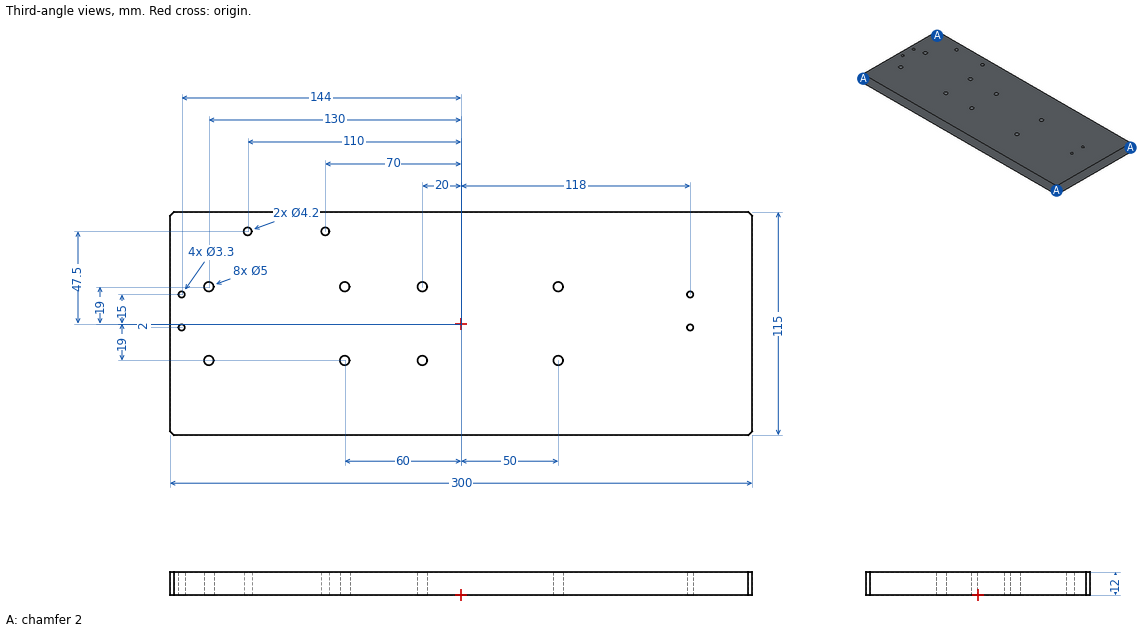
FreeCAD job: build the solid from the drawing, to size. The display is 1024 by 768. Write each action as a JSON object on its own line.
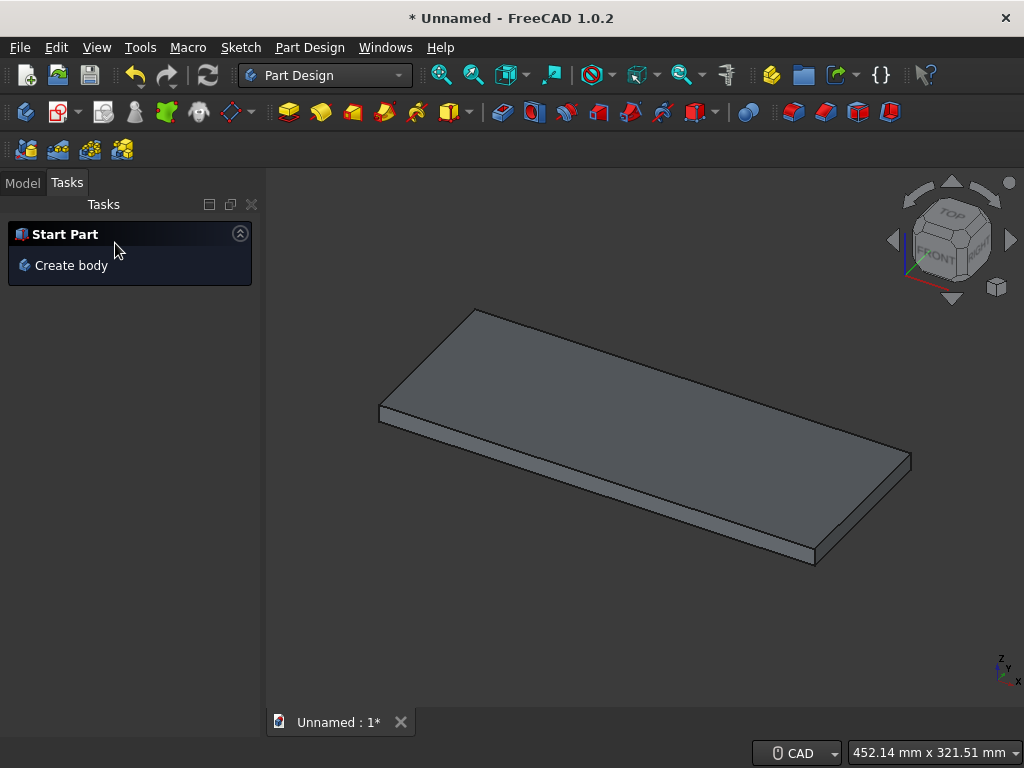
{"action": "left_click", "coordinate": [58, 112]}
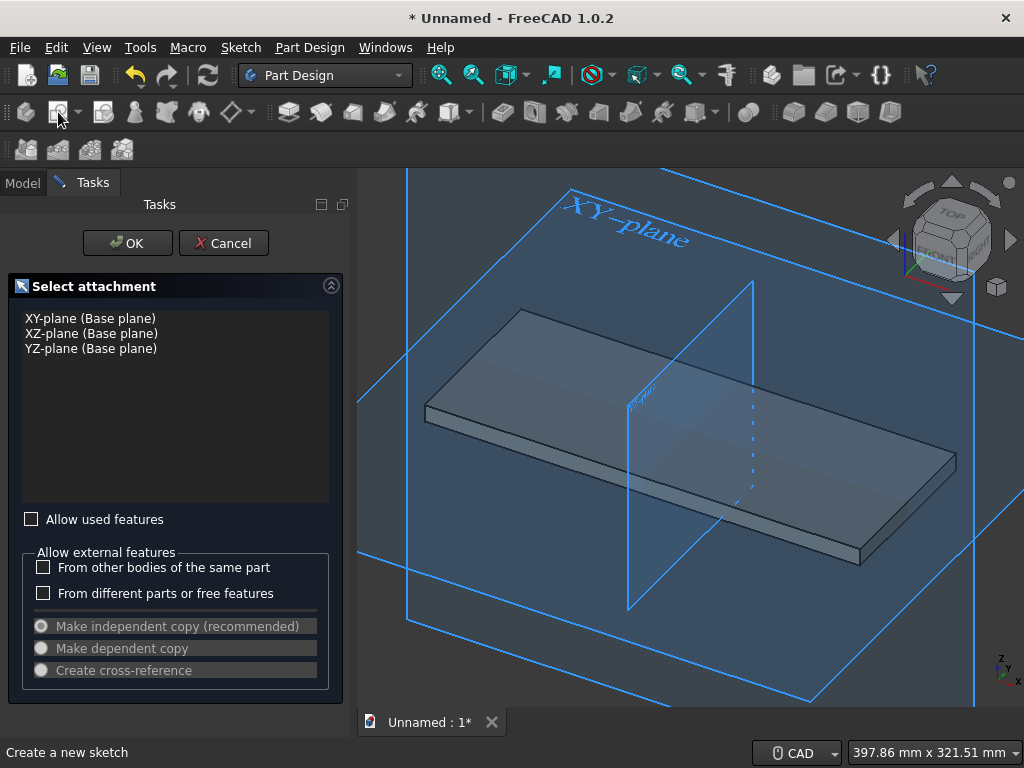
{"action": "left_click", "coordinate": [82, 318]}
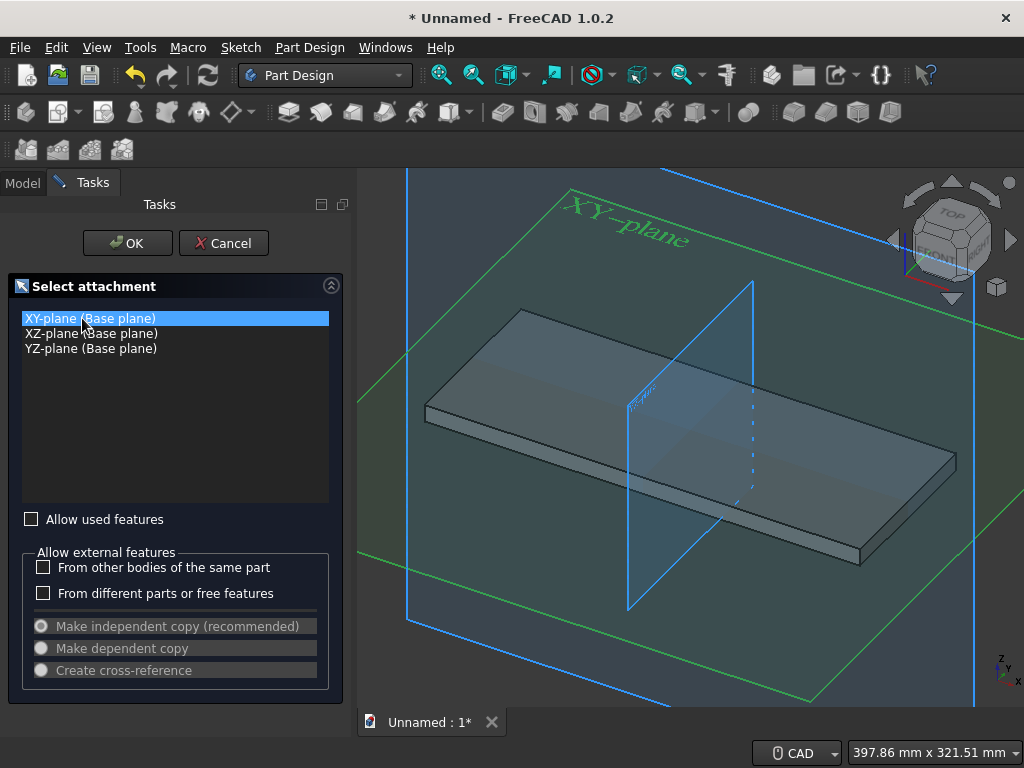
{"action": "left_click", "coordinate": [128, 243]}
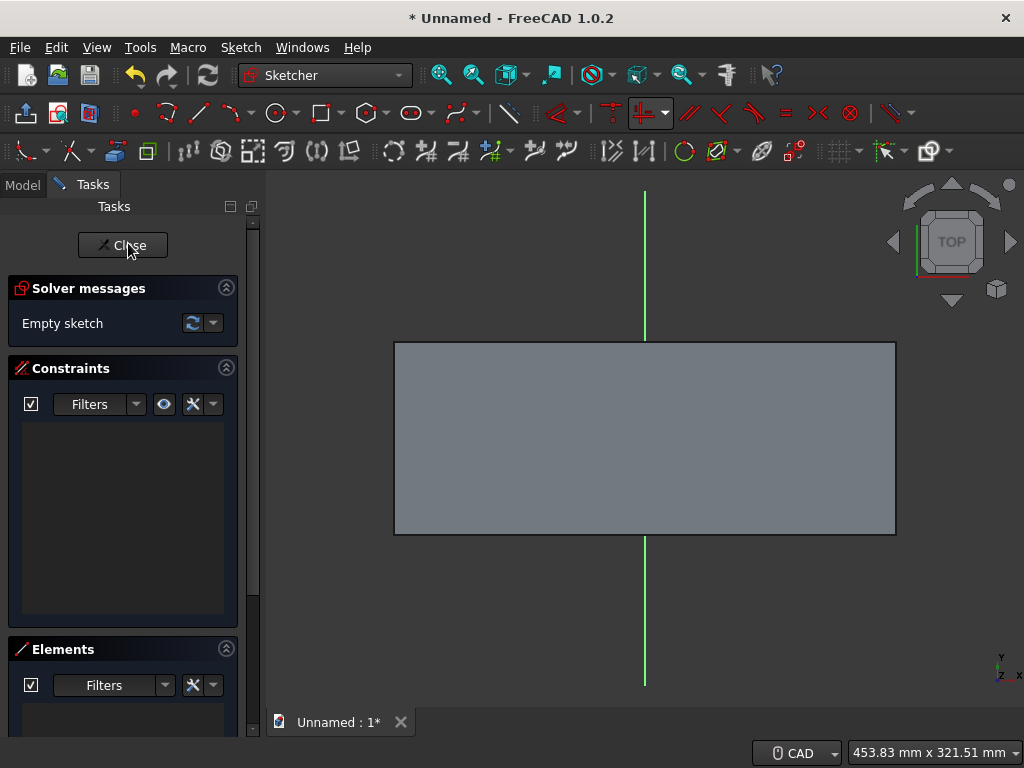
{"action": "left_click", "coordinate": [90, 114]}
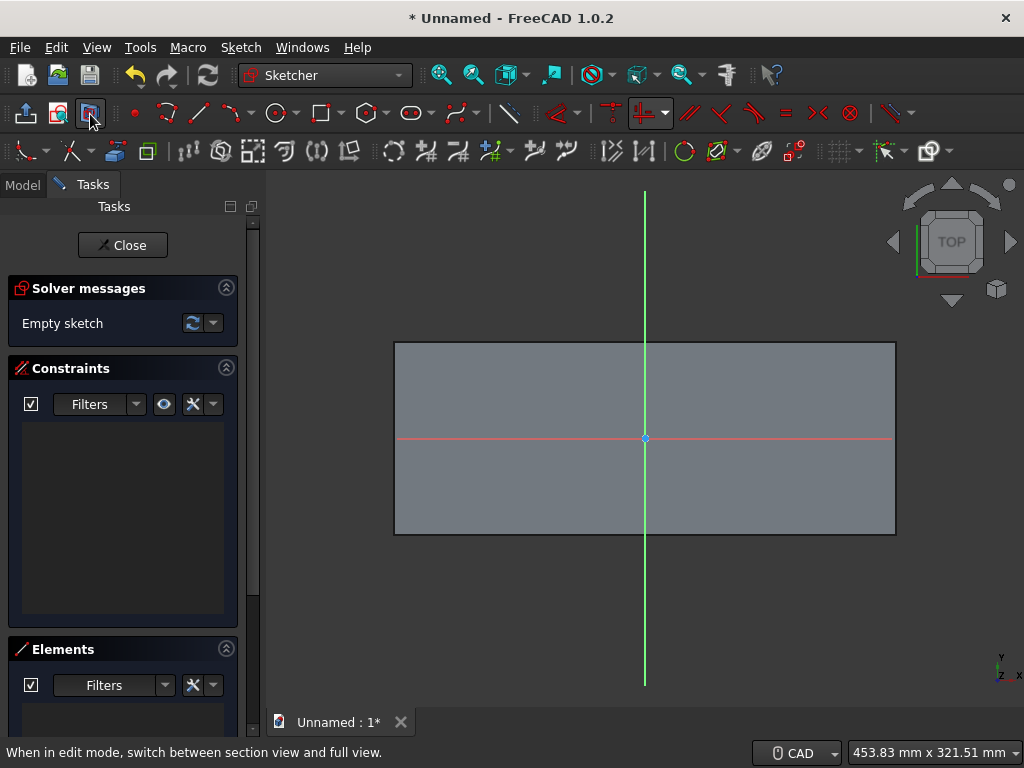
{"action": "left_click", "coordinate": [276, 114]}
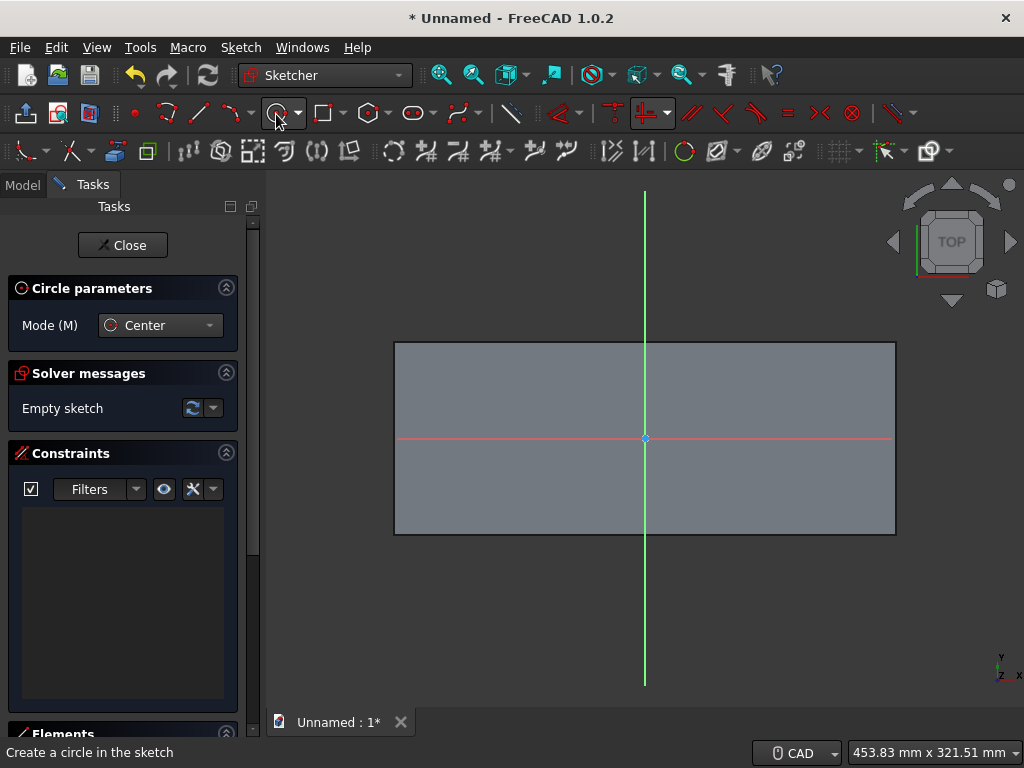
{"action": "scroll", "coordinate": [428, 407], "scroll_direction": "up", "scroll_amount": 9}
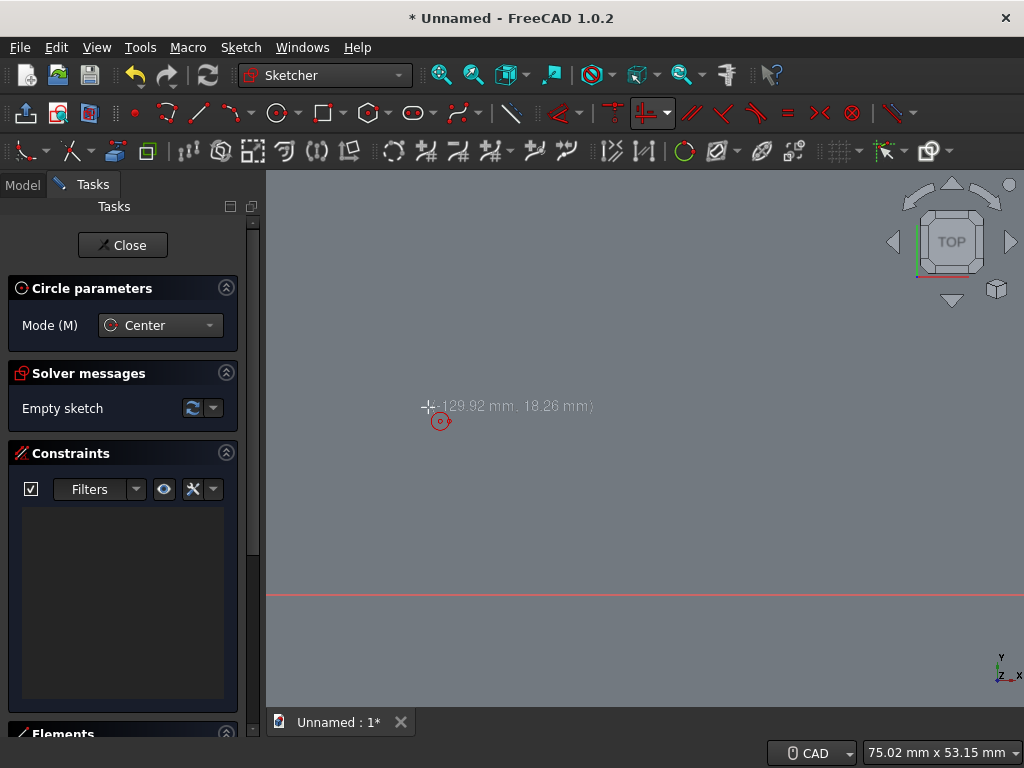
{"action": "scroll", "coordinate": [384, 399], "scroll_direction": "down", "scroll_amount": 8}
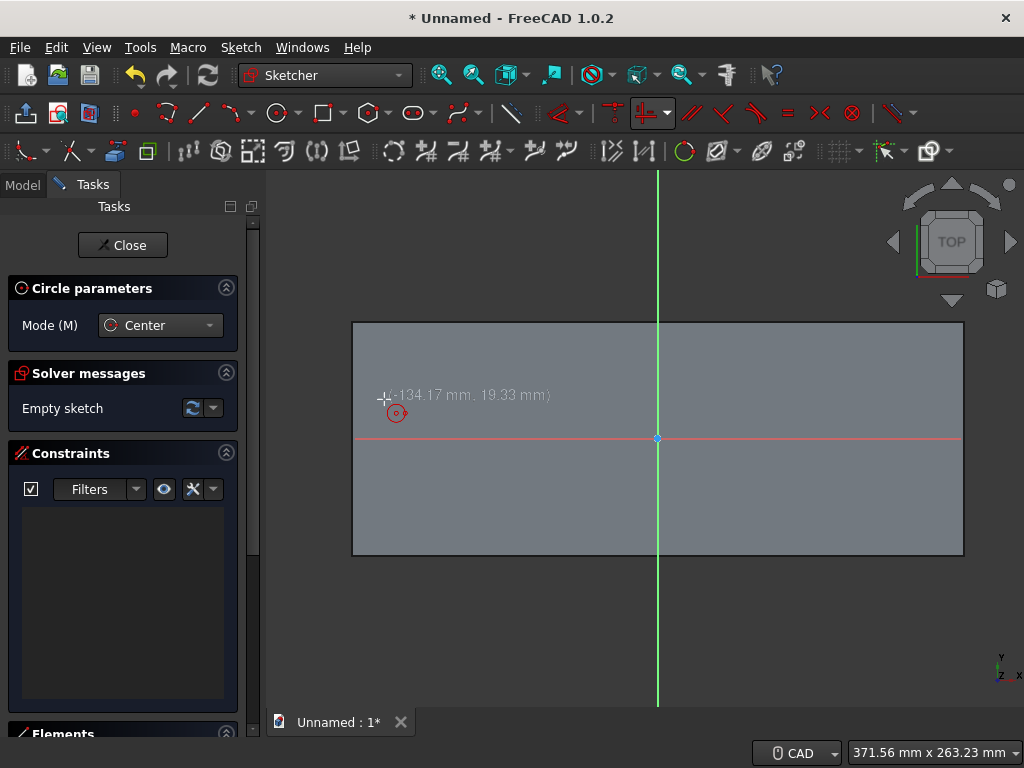
{"action": "left_click", "coordinate": [393, 400]}
{"action": "mouse_move", "coordinate": [396, 397]}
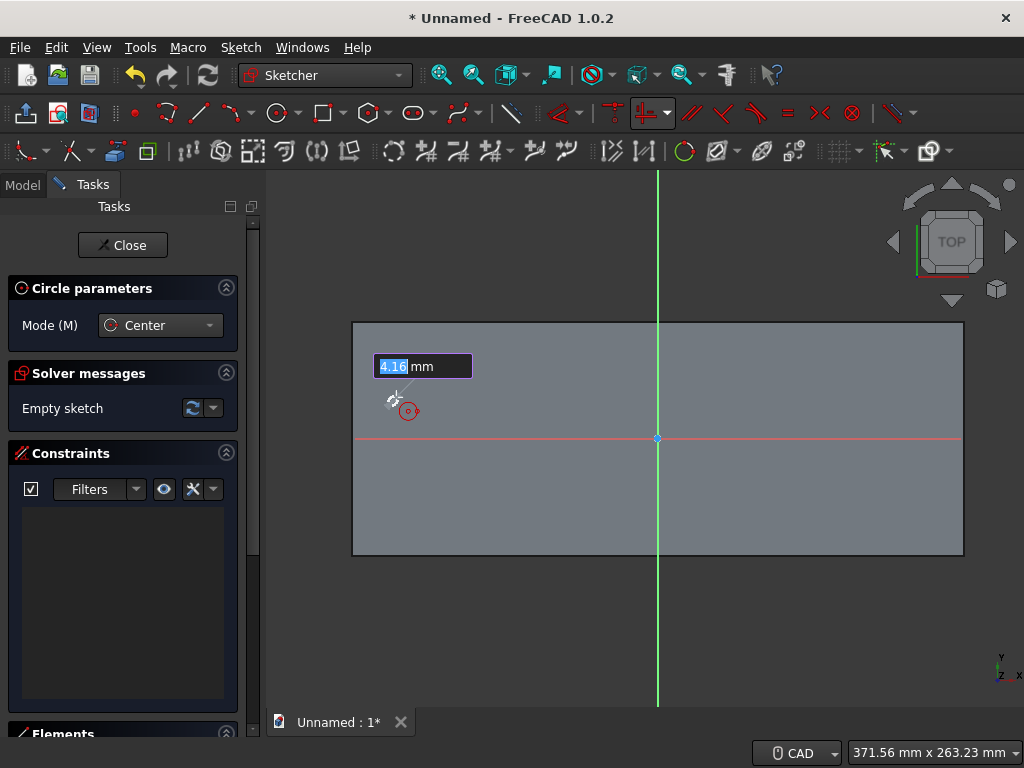
{"action": "type", "text": "5"}
{"action": "key", "text": "Return"}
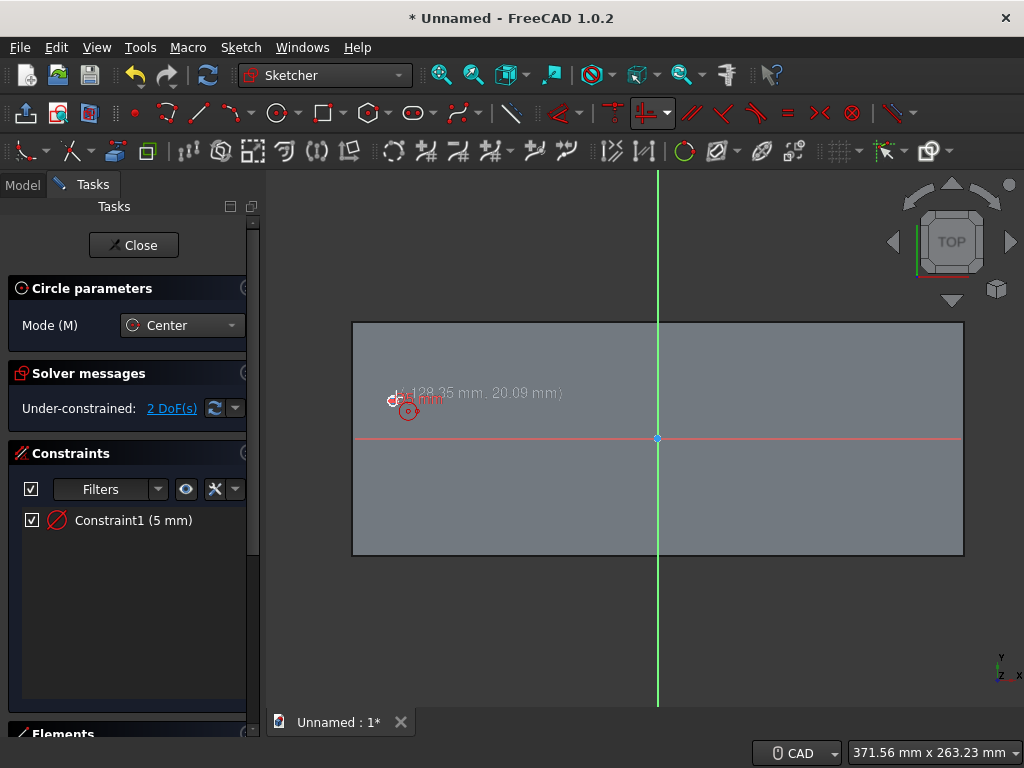
{"action": "scroll", "coordinate": [535, 478], "scroll_direction": "up", "scroll_amount": 8}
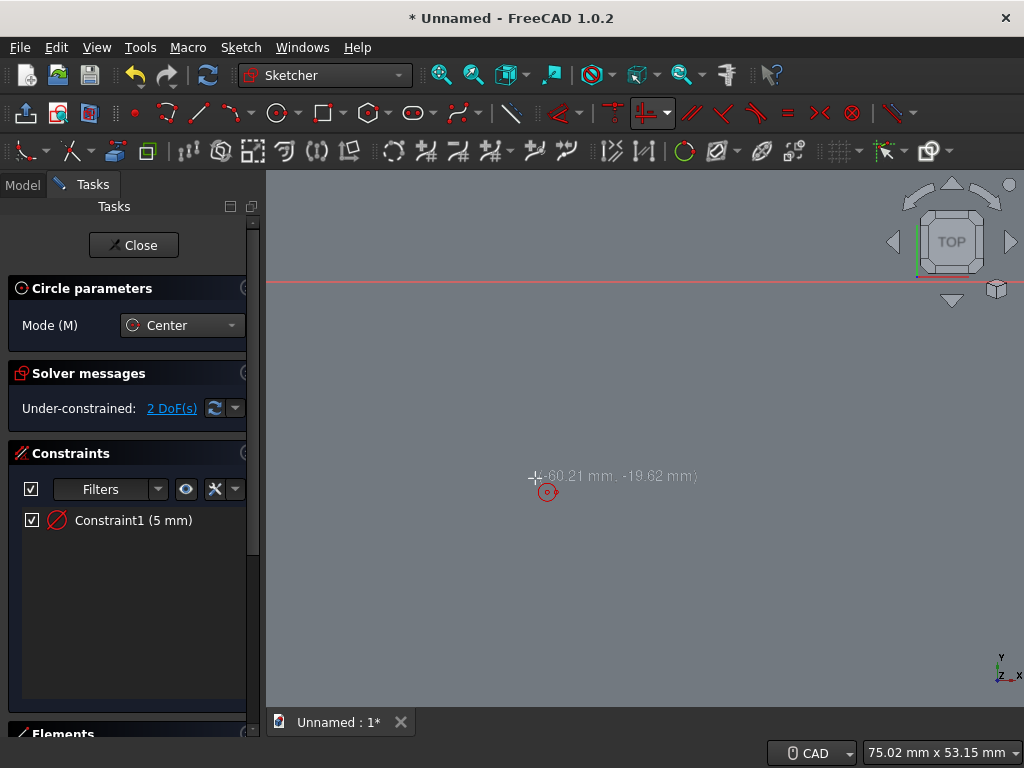
{"action": "scroll", "coordinate": [536, 478], "scroll_direction": "down", "scroll_amount": 8}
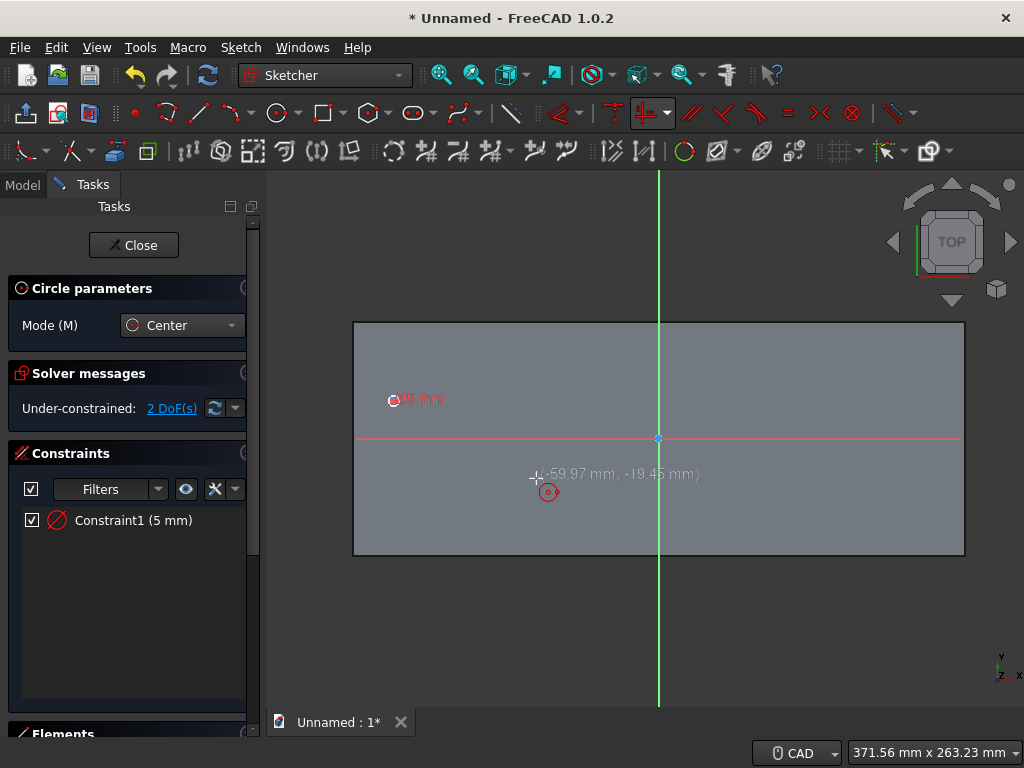
{"action": "left_click", "coordinate": [536, 478]}
{"action": "mouse_move", "coordinate": [540, 474]}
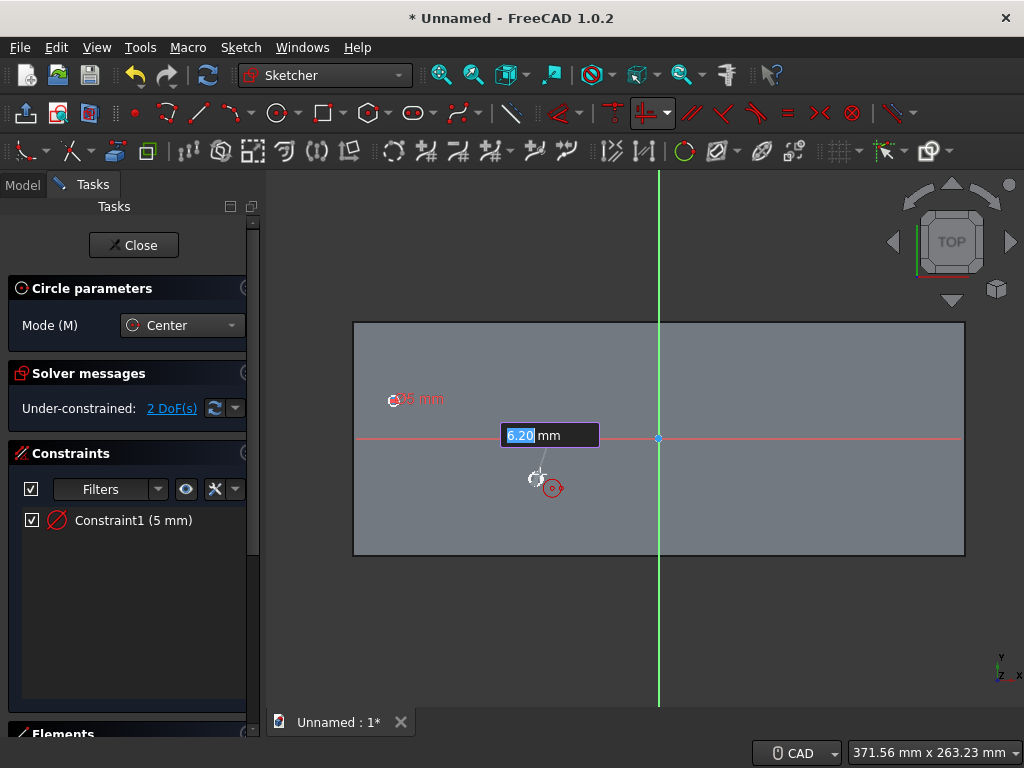
{"action": "type", "text": "5"}
{"action": "key", "text": "Return"}